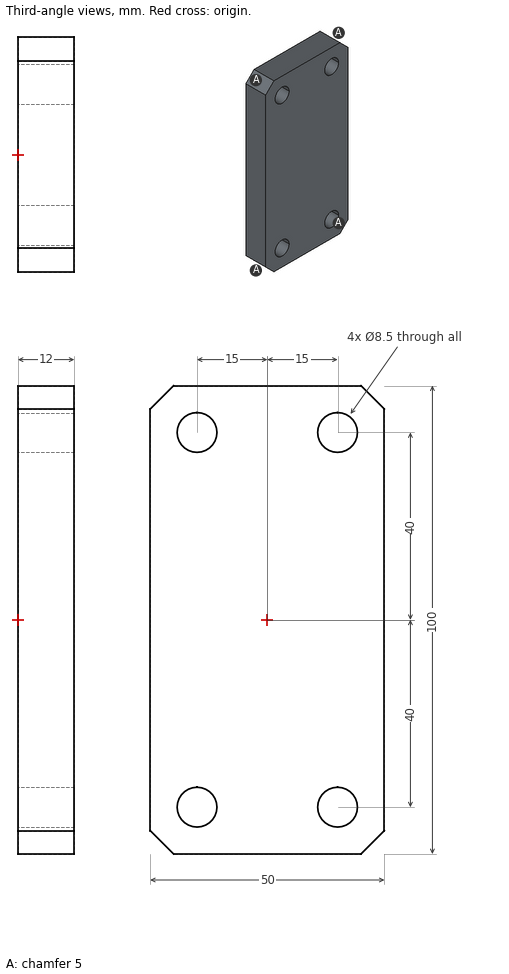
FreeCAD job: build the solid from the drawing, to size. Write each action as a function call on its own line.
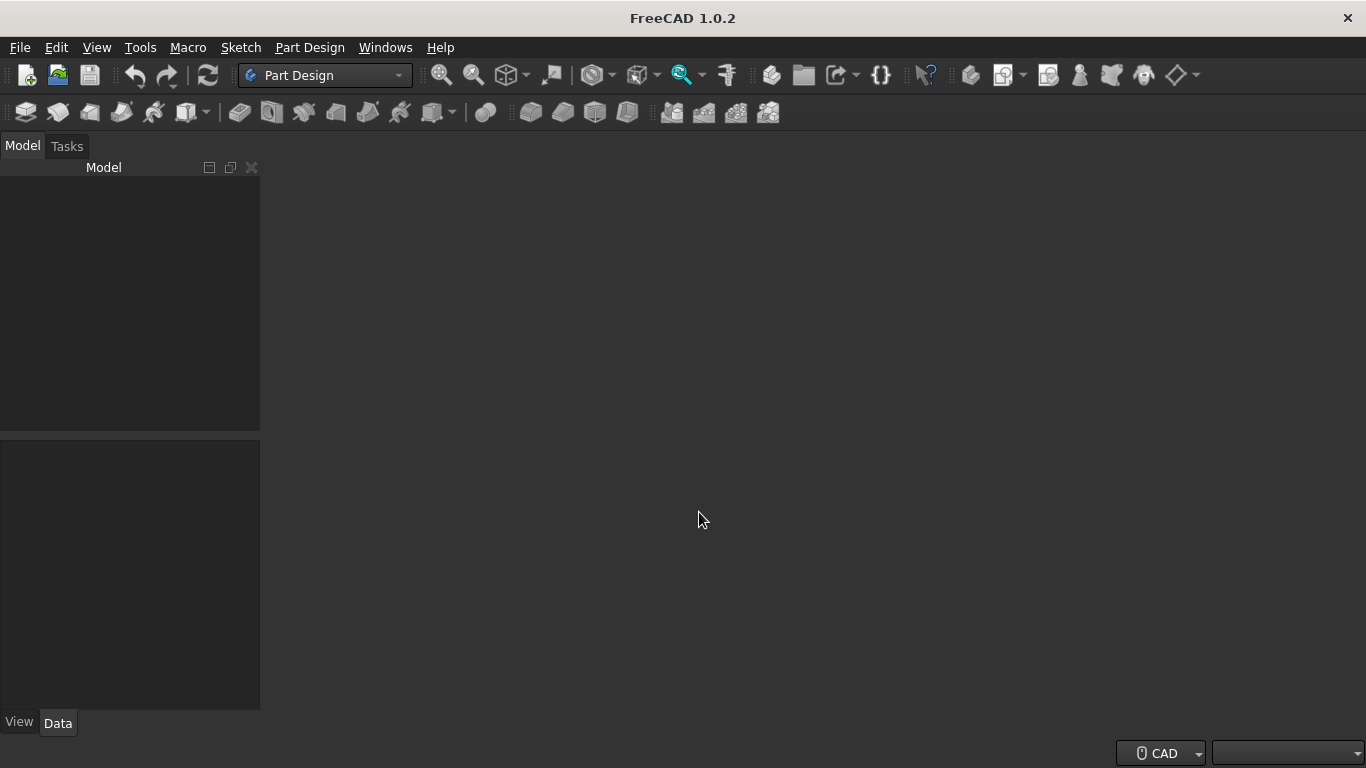
click(26, 76)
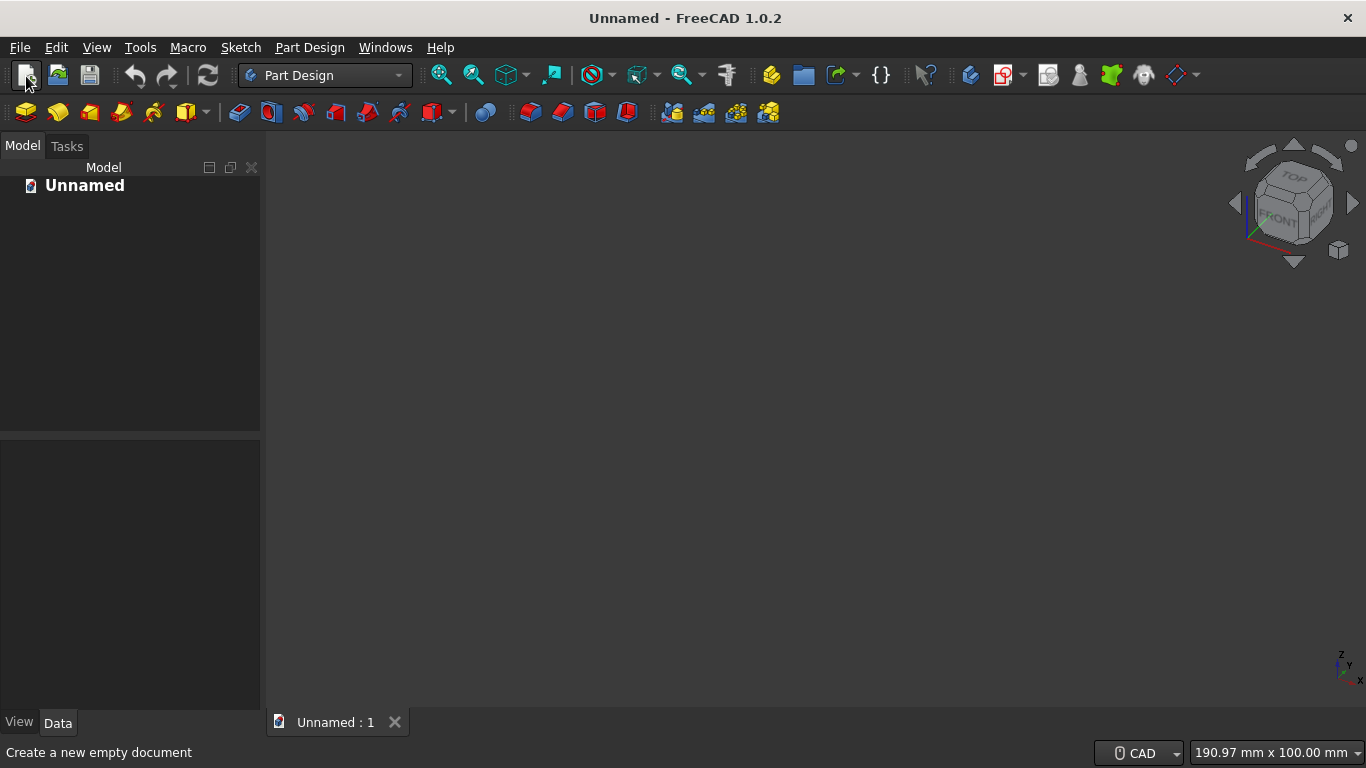
click(1004, 76)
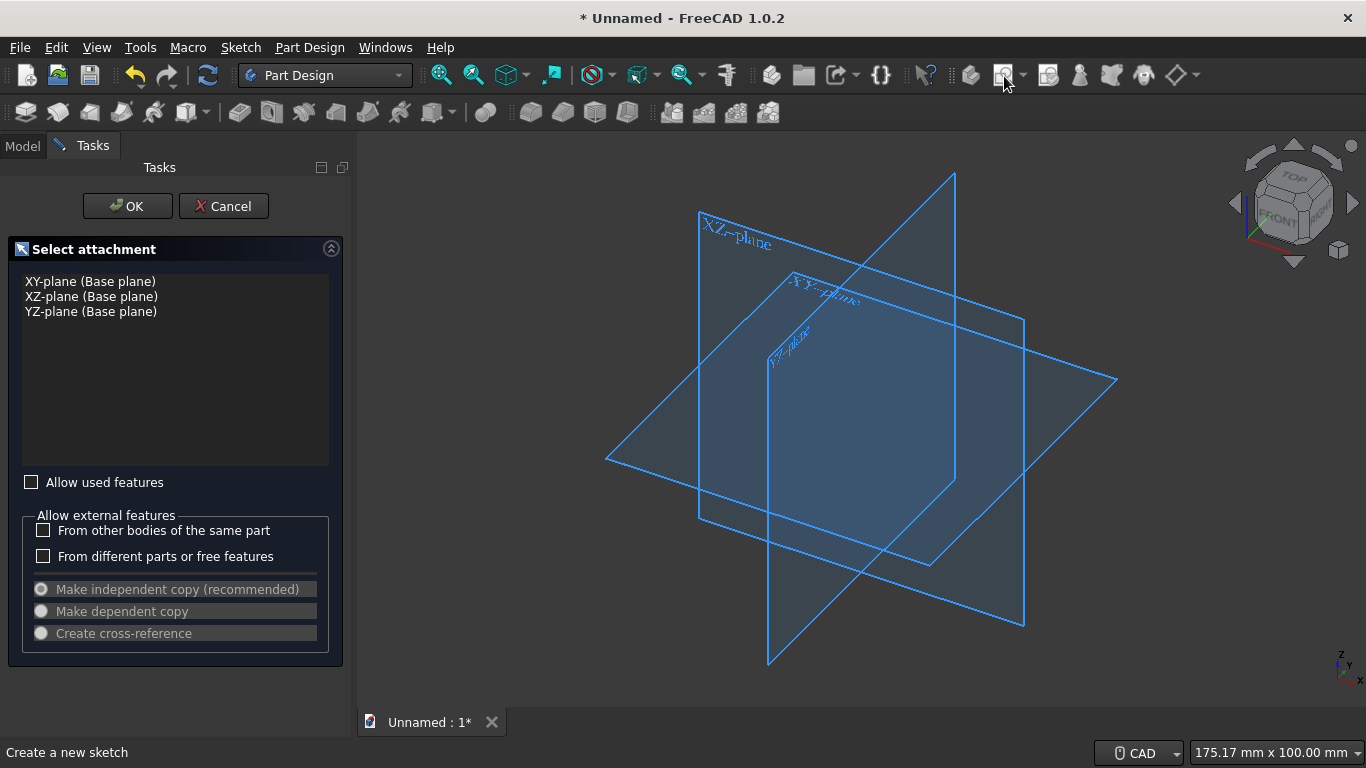
click(82, 312)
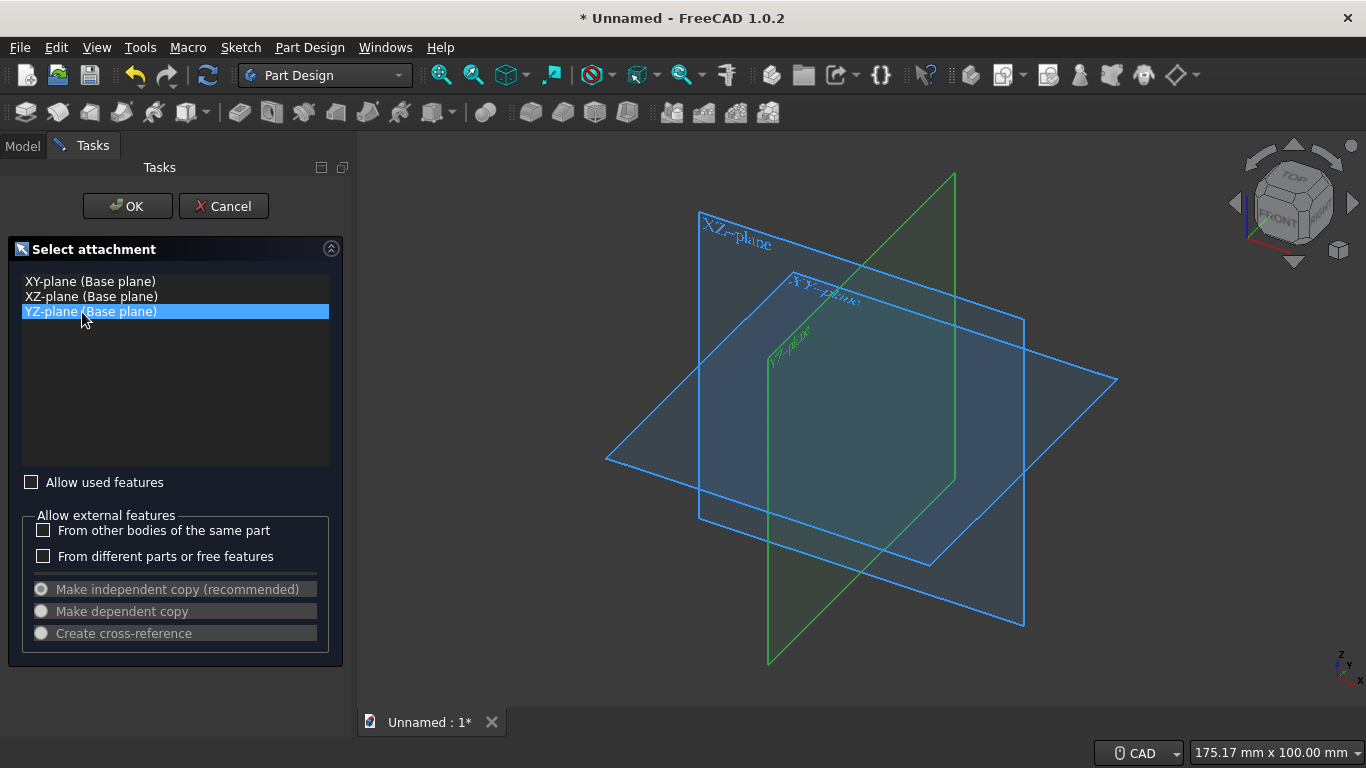
click(128, 206)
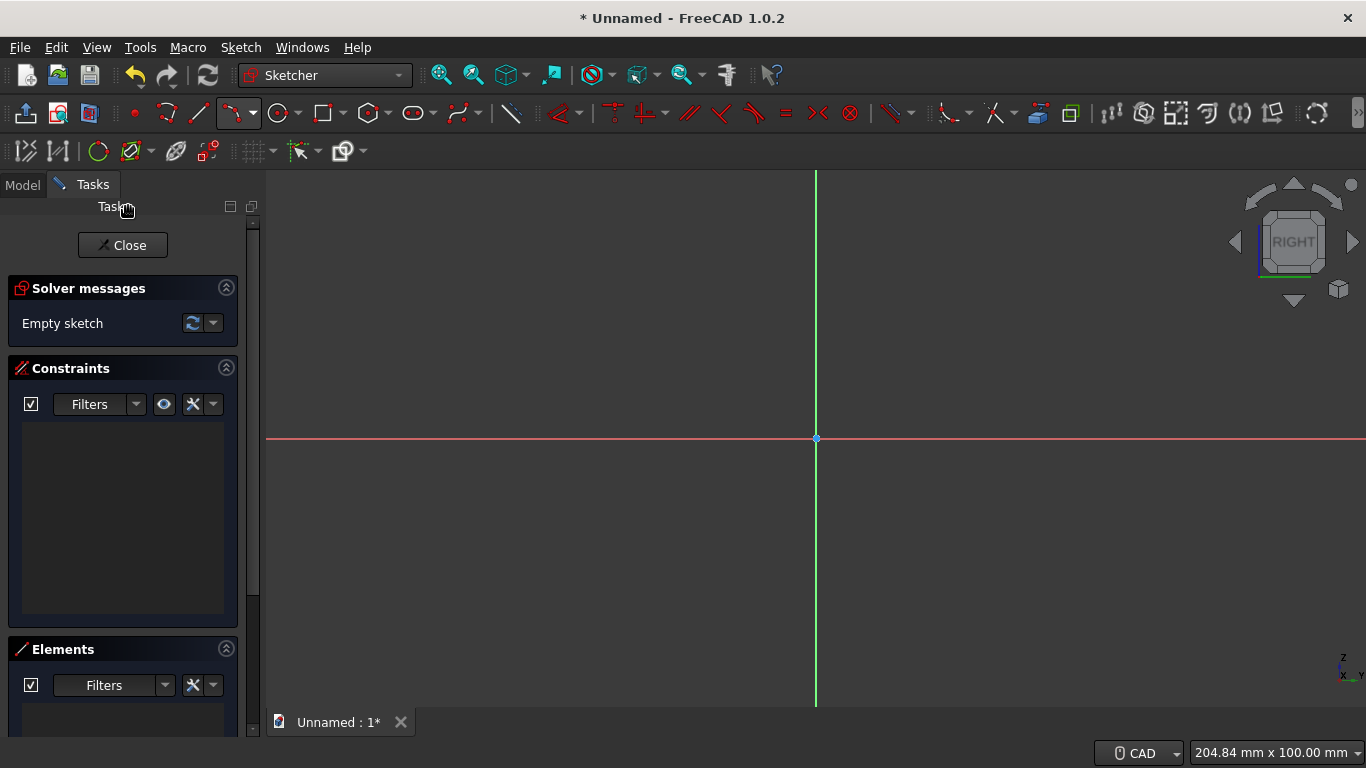
scroll(608, 438, down, 2)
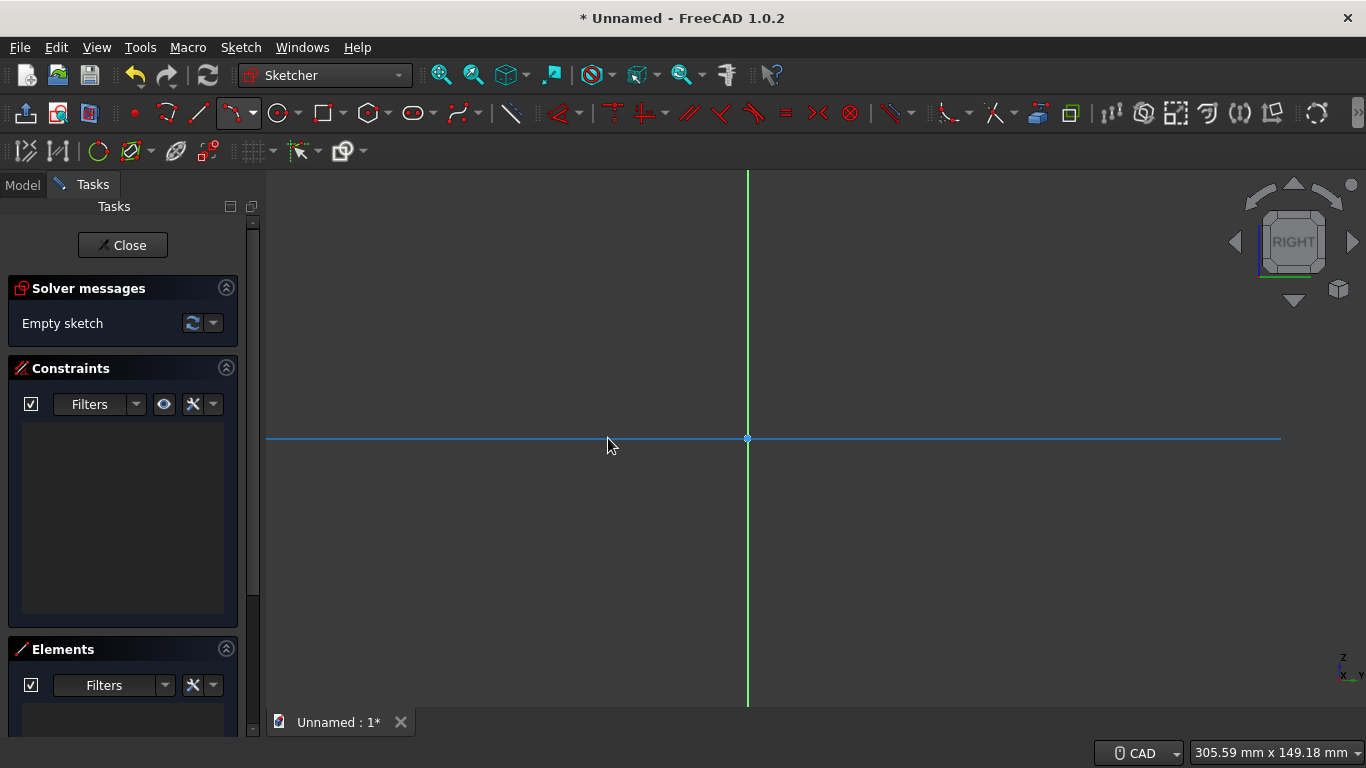
key(g)
key(v)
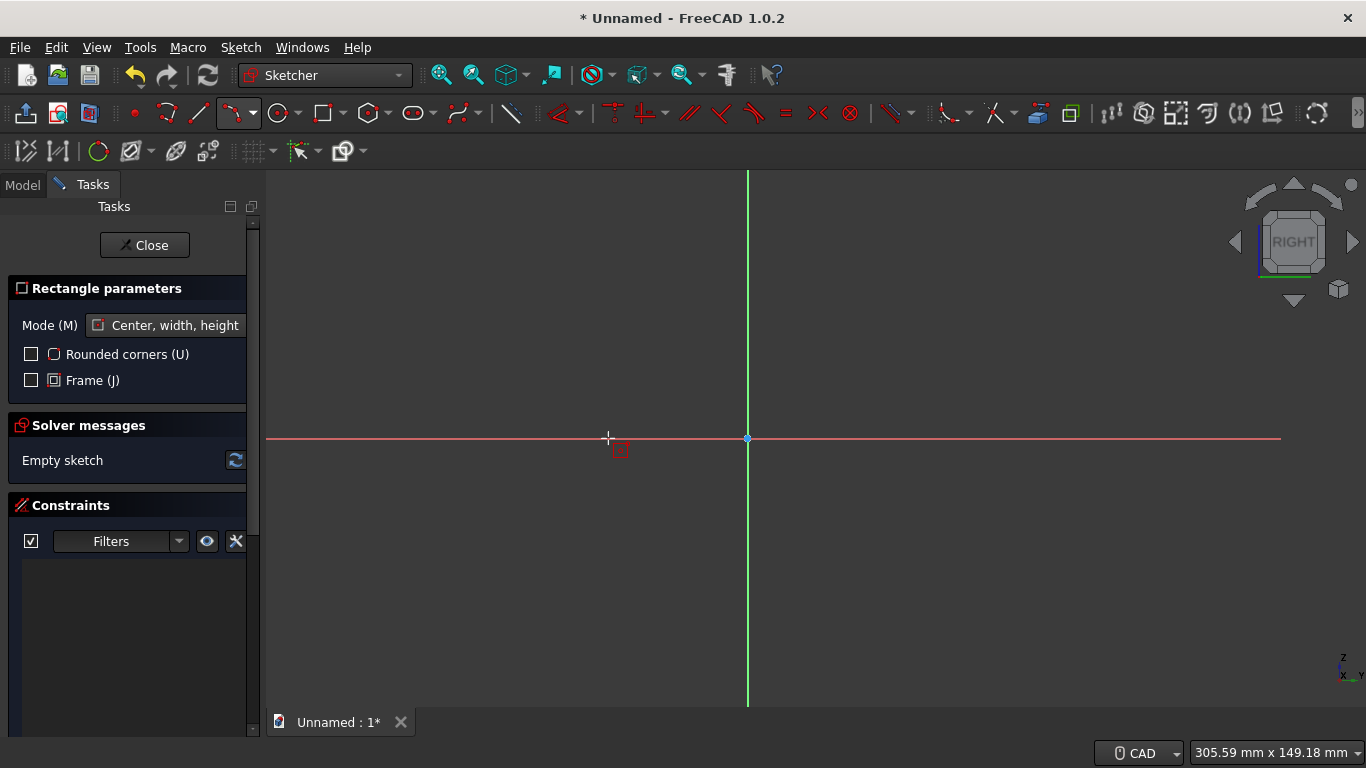
click(748, 438)
move(838, 259)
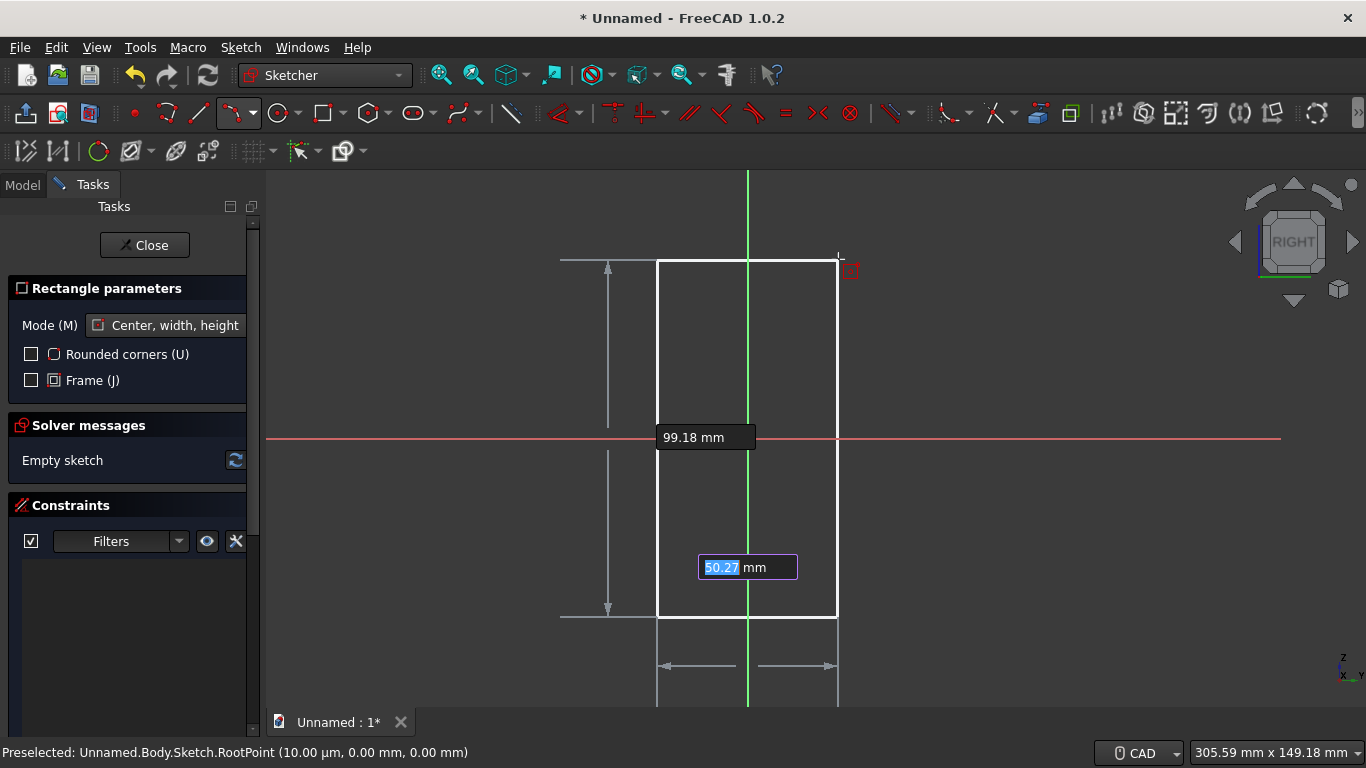
text(50)
key(Tab)
text(100)
key(Return)
key(Escape)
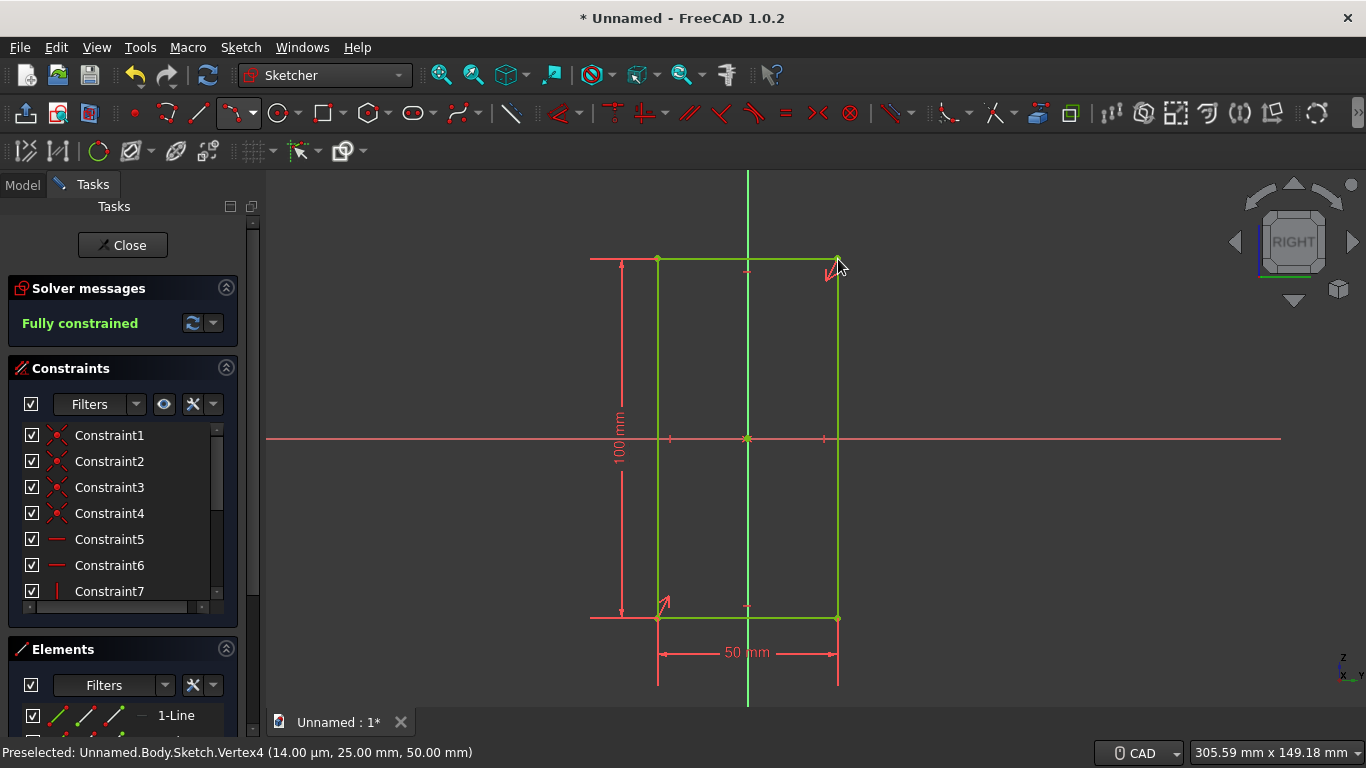
click(123, 245)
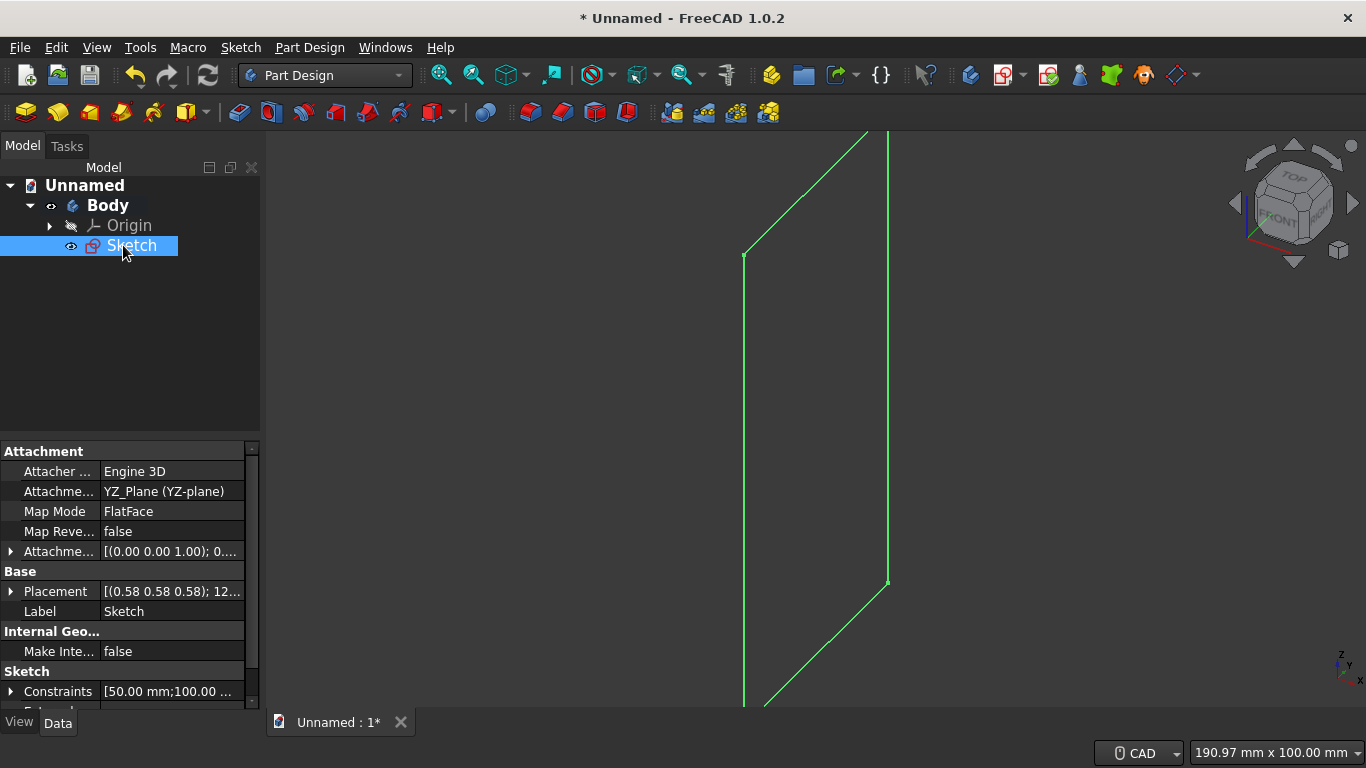
click(26, 112)